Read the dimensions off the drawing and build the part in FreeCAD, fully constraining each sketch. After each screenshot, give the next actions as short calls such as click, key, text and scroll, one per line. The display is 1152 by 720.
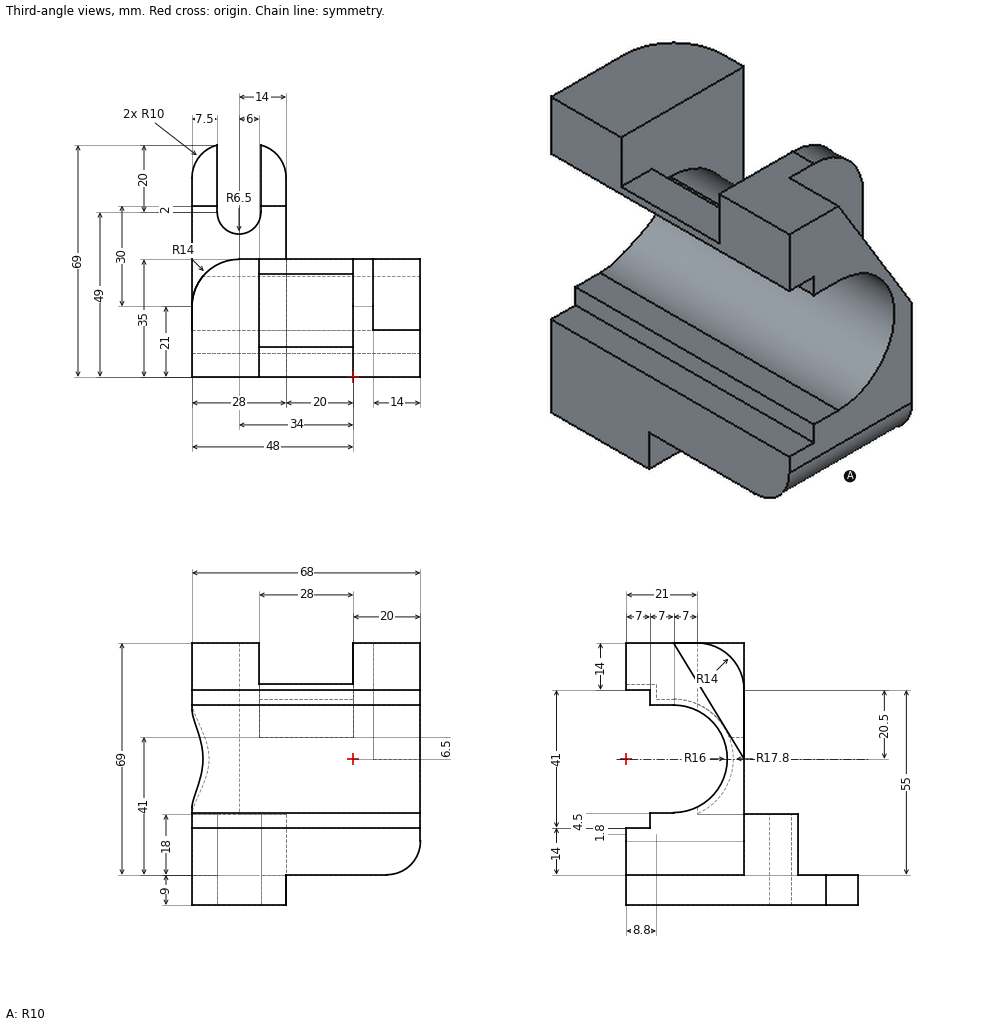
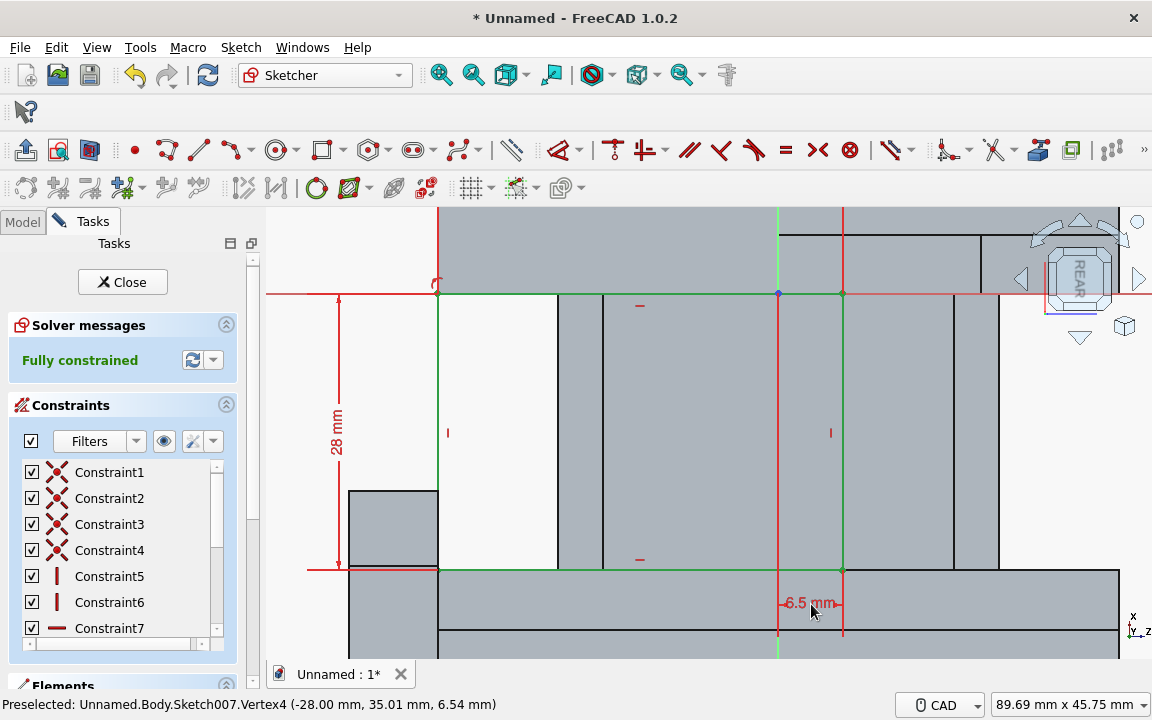
click(123, 282)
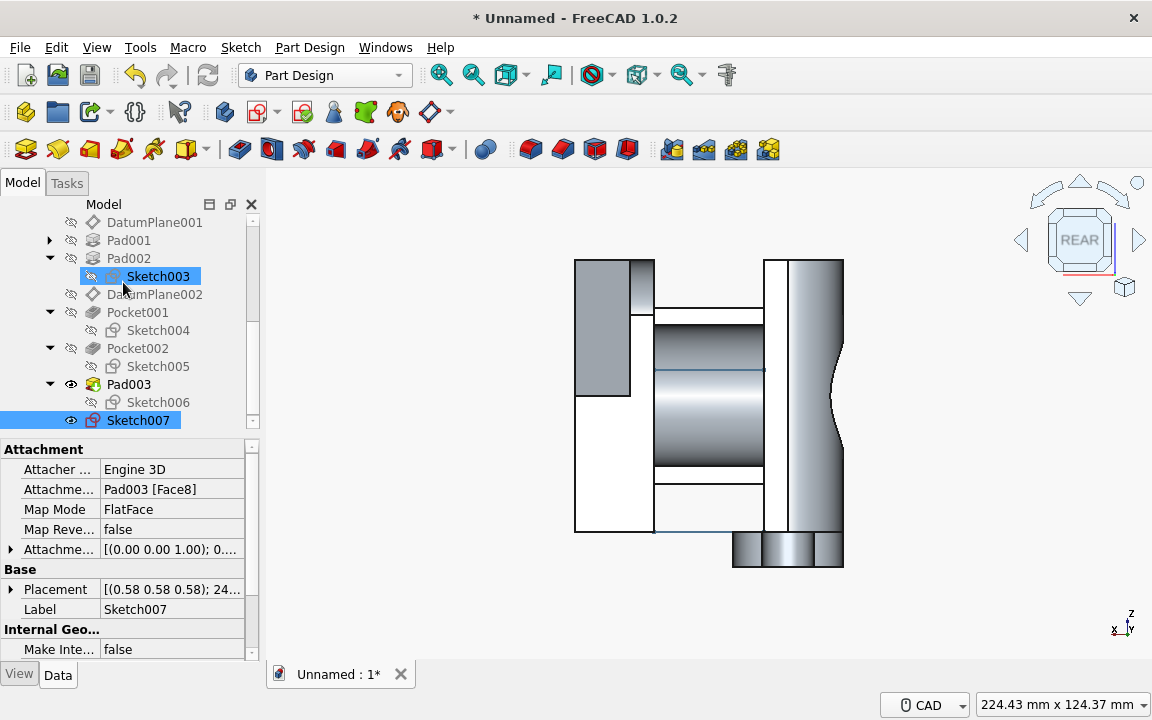
click(26, 150)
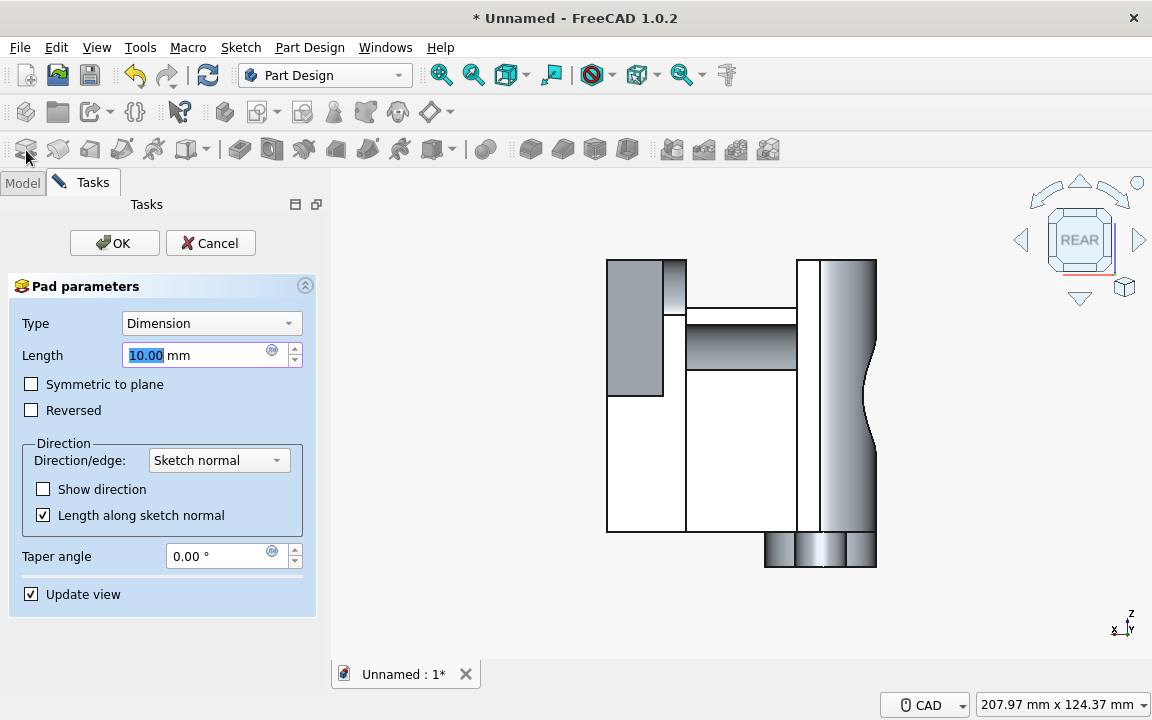
text(35)
key(Tab)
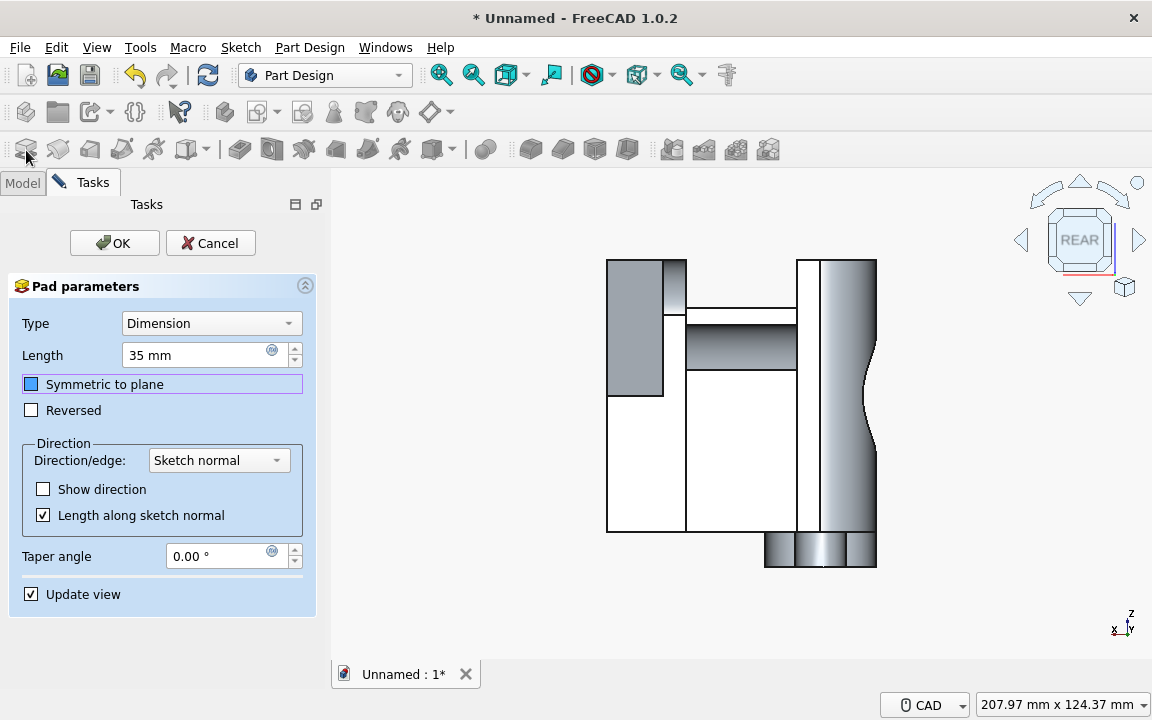
click(30, 410)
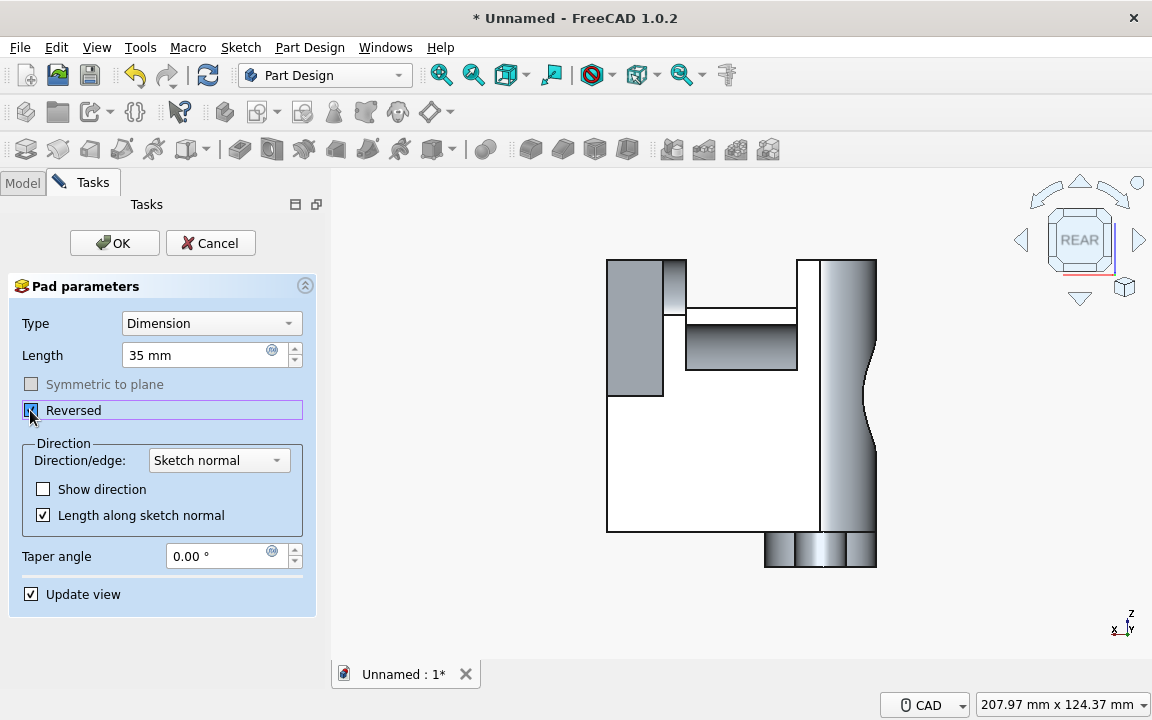
click(115, 243)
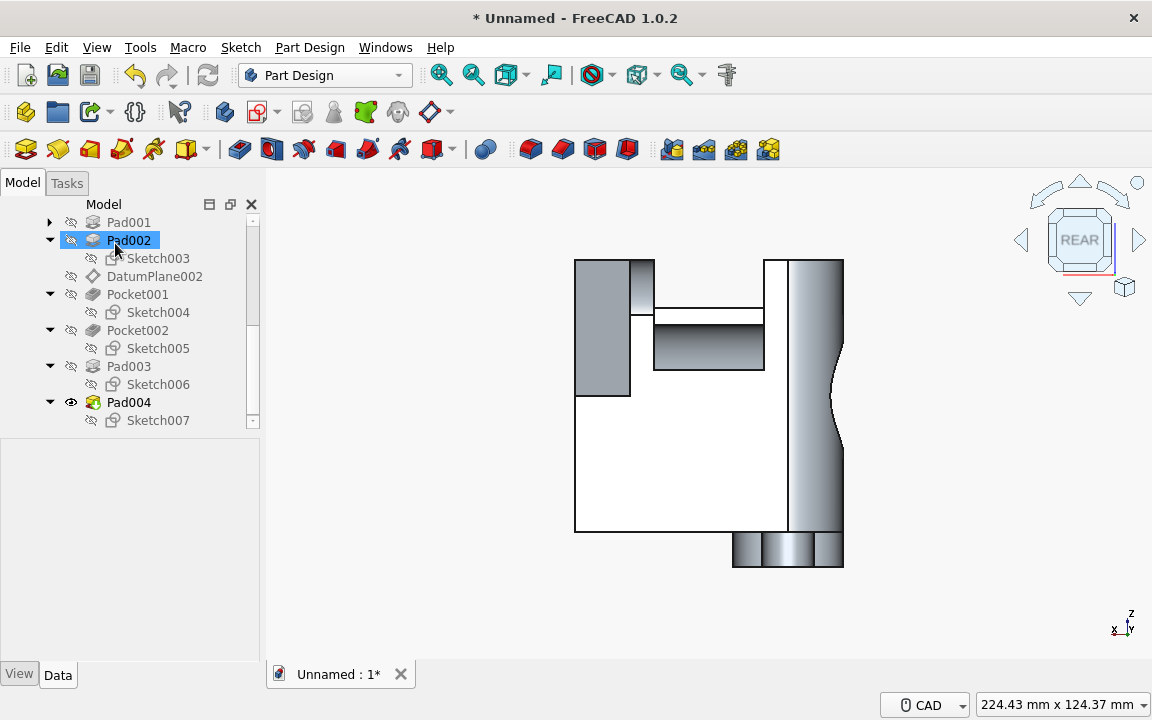
scroll(140, 326, down, 3)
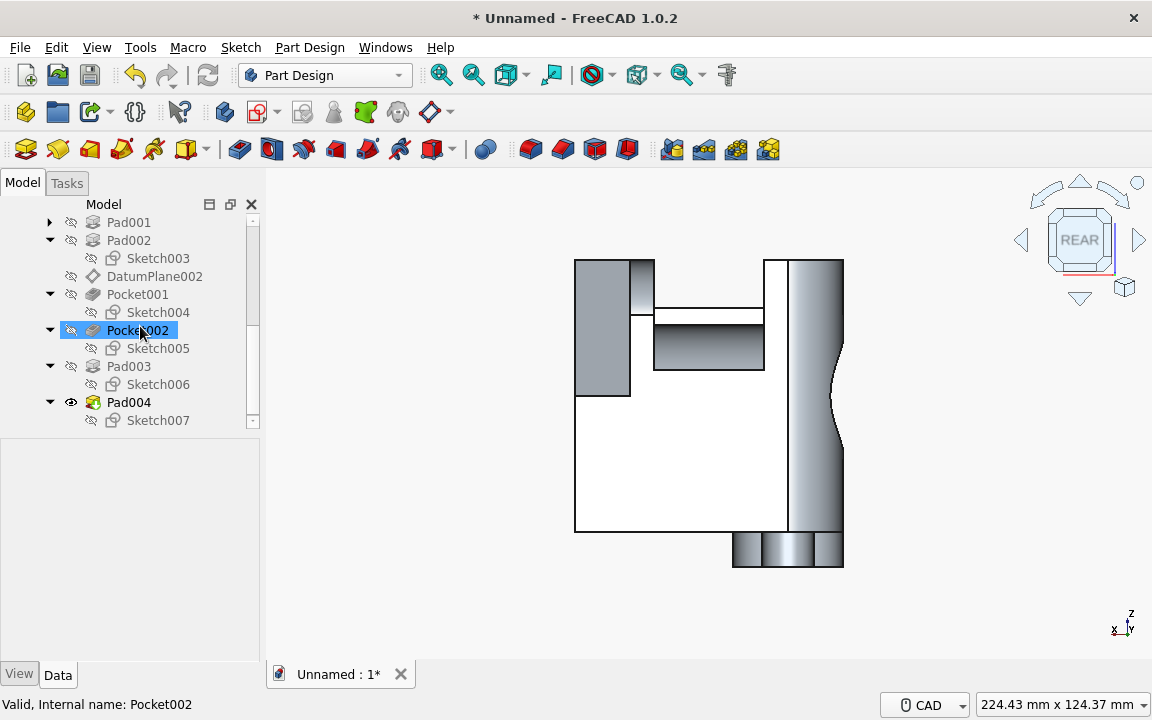
scroll(140, 326, up, 15)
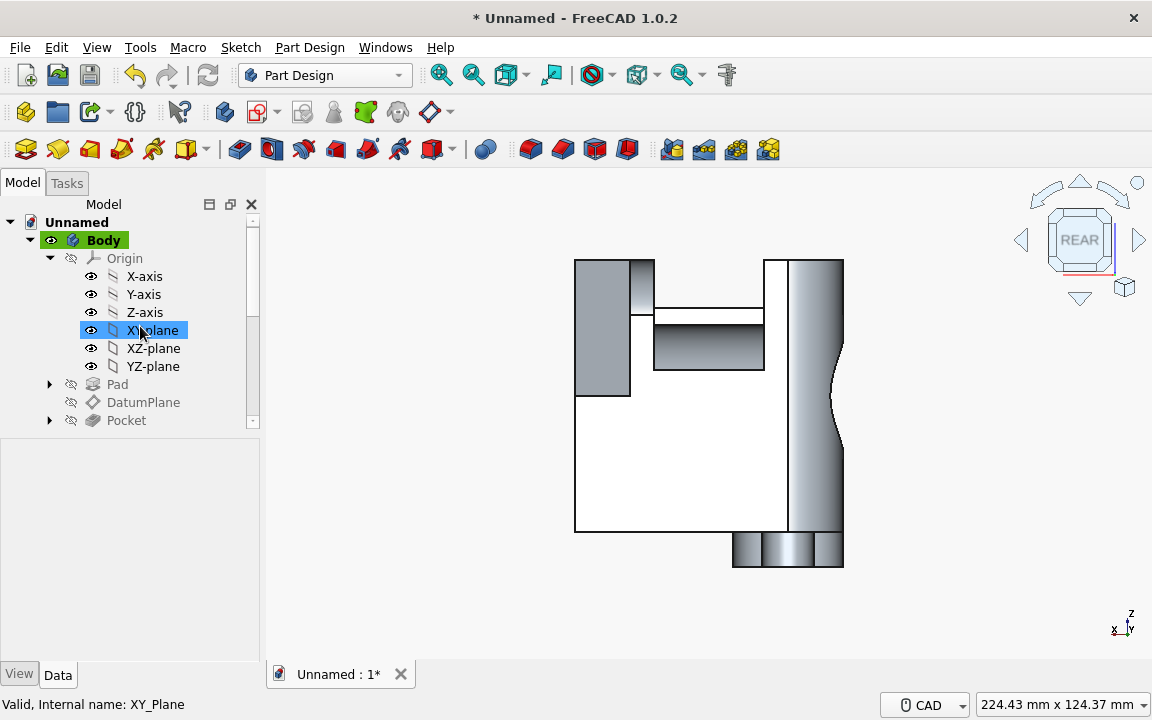
click(136, 366)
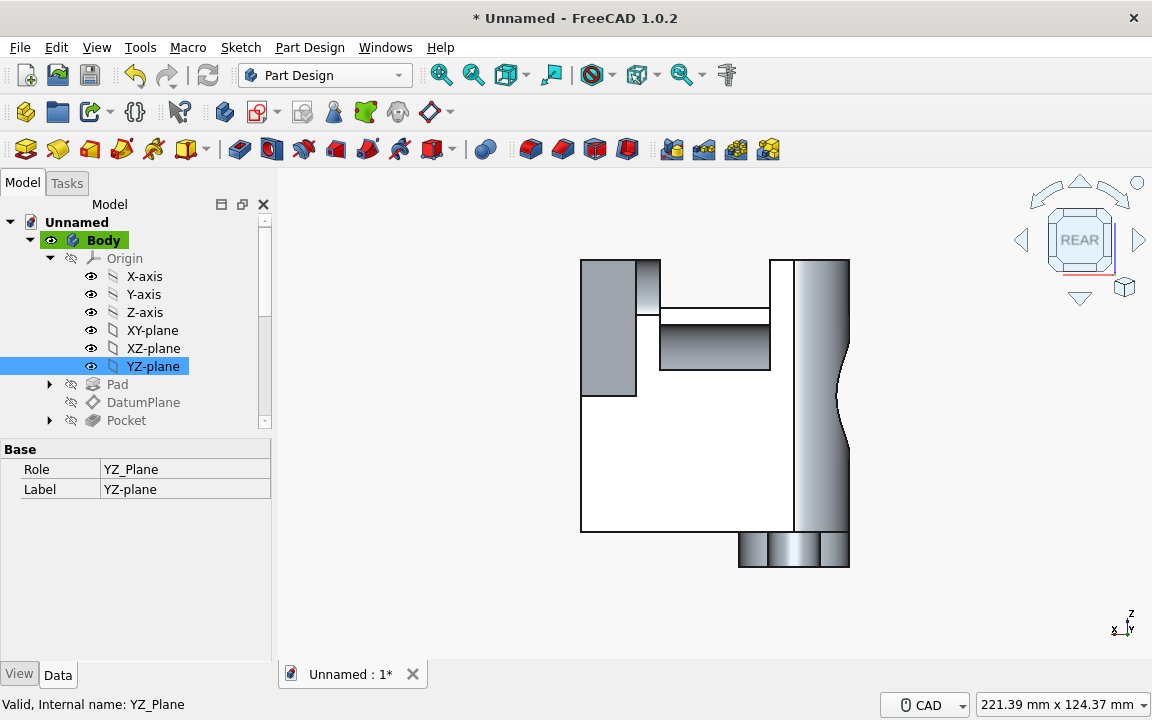
click(430, 112)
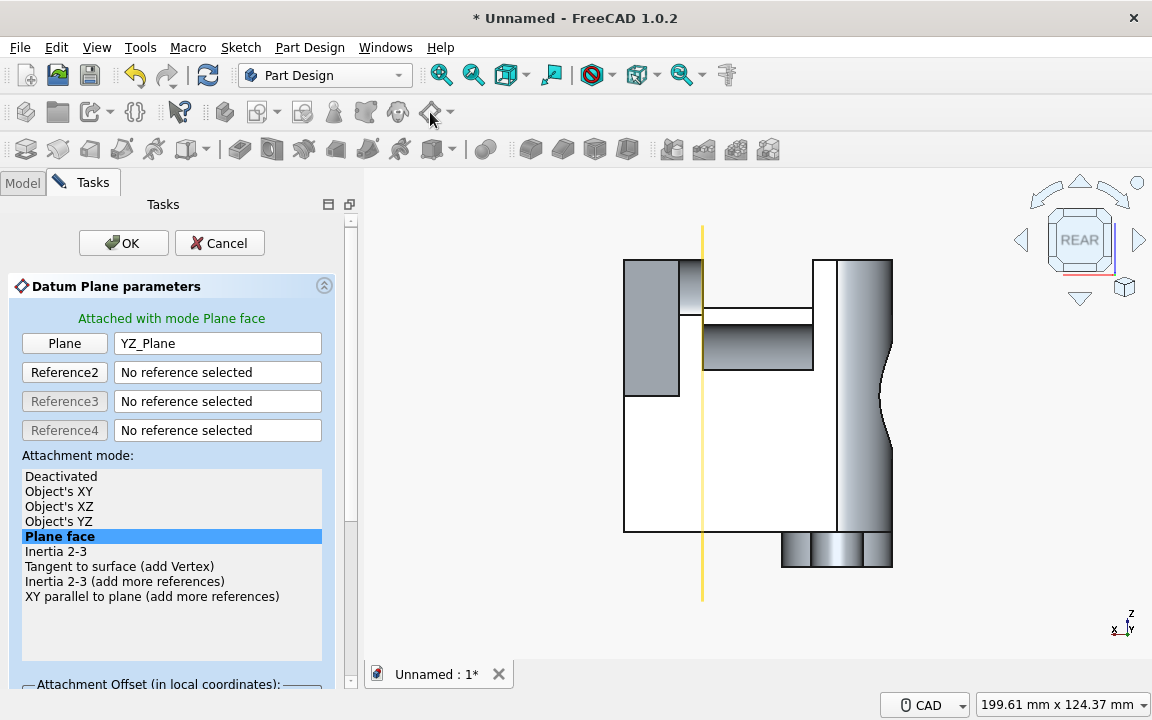
scroll(351, 451, down, 3)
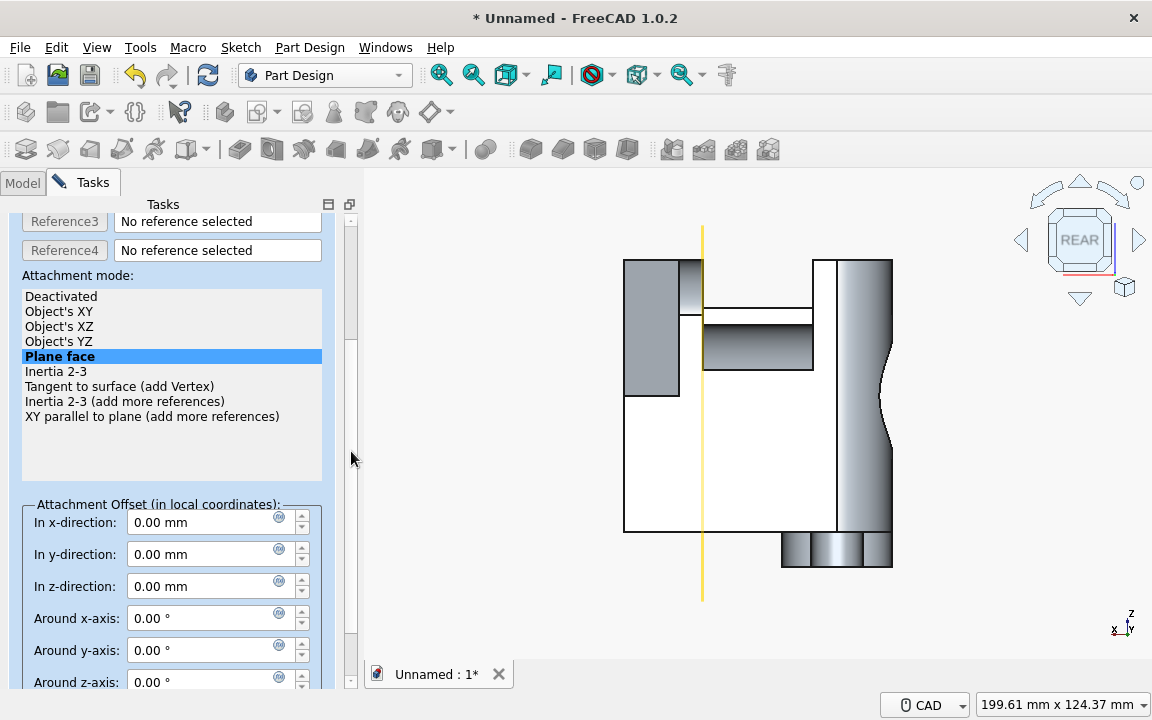
triple_click(210, 586)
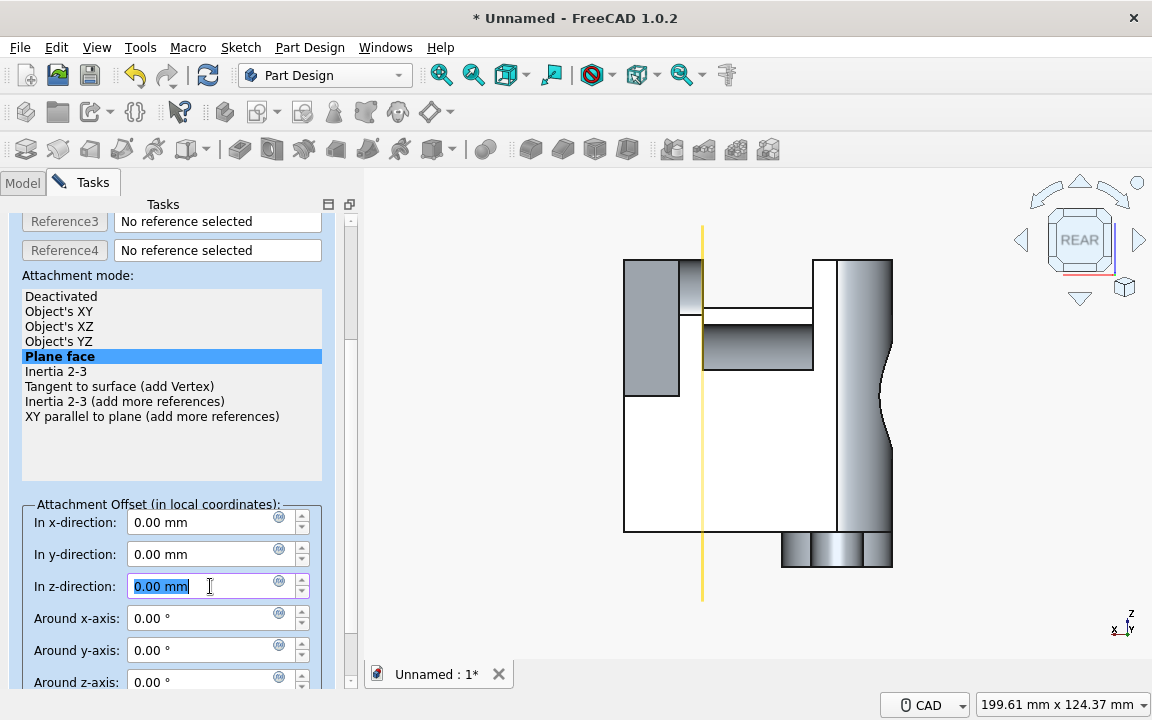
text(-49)
key(Tab)